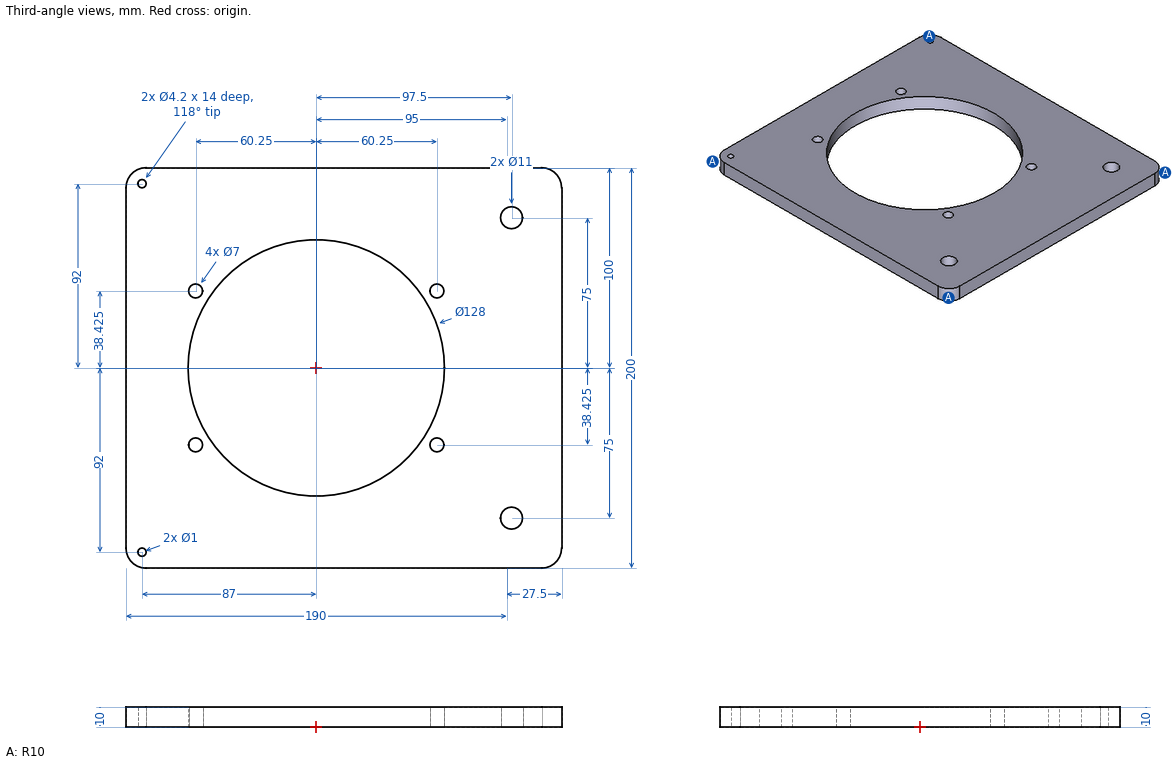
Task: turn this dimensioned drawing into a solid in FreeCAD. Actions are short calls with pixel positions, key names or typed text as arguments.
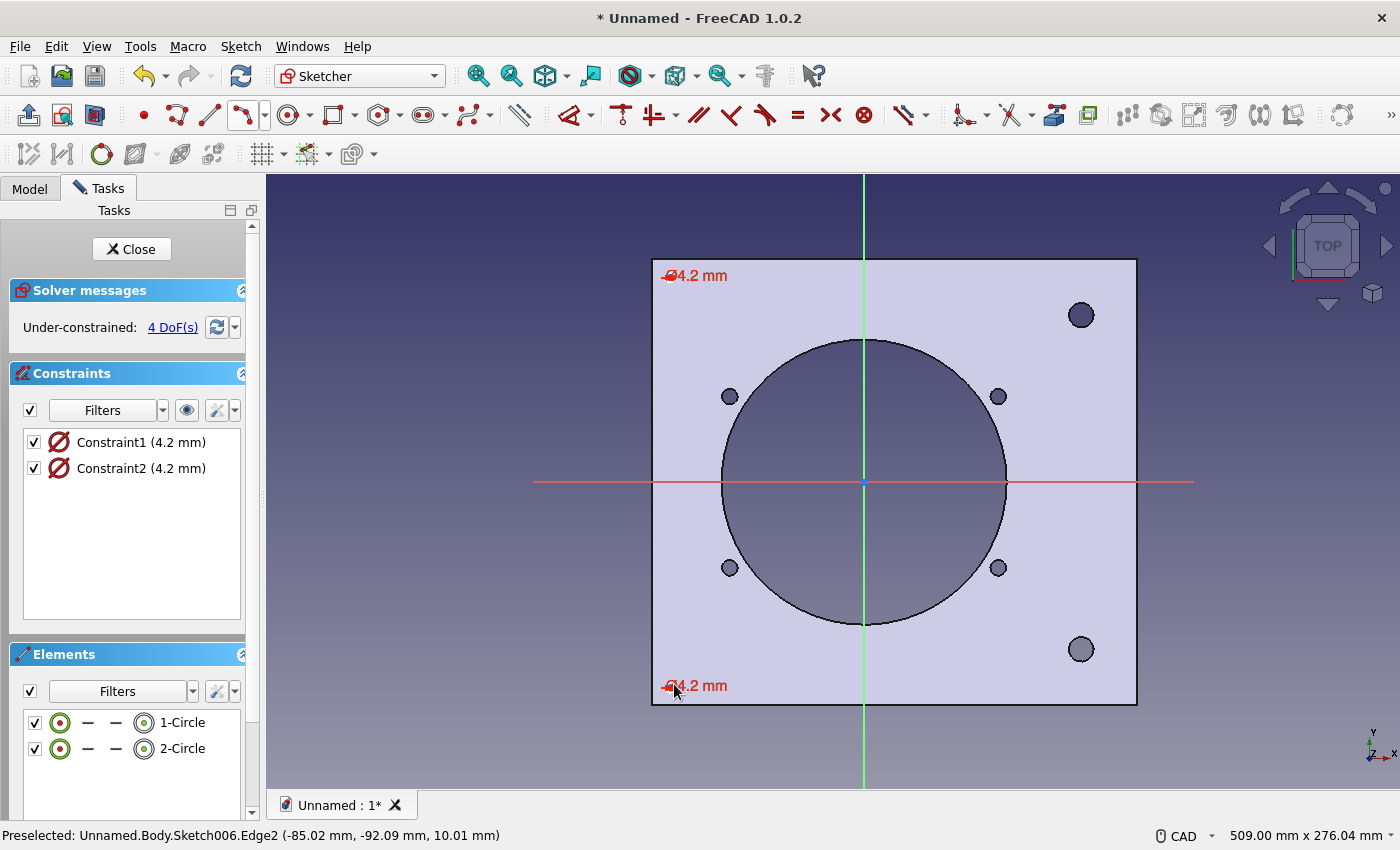
click(670, 278)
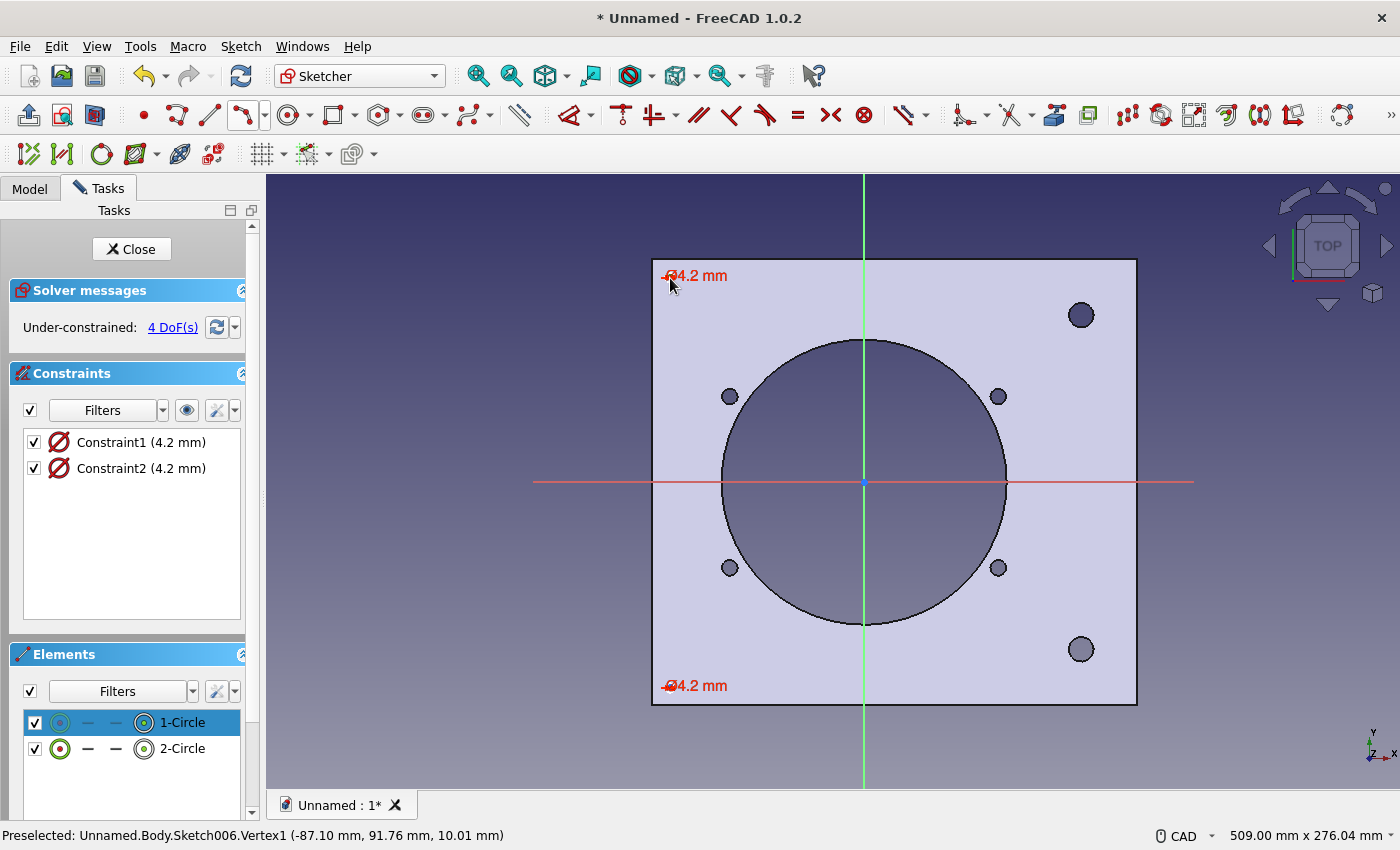
click(670, 688)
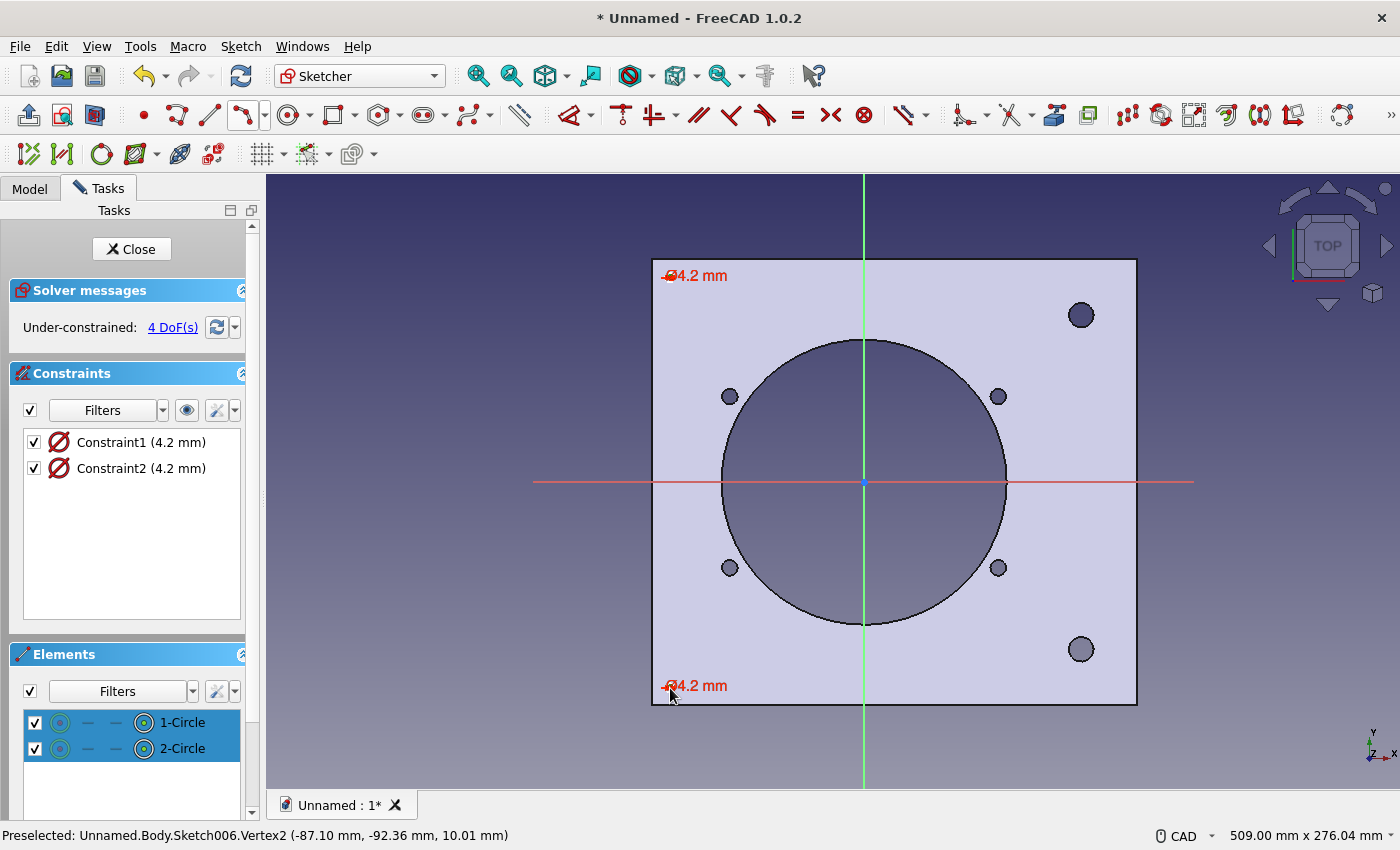
key(v)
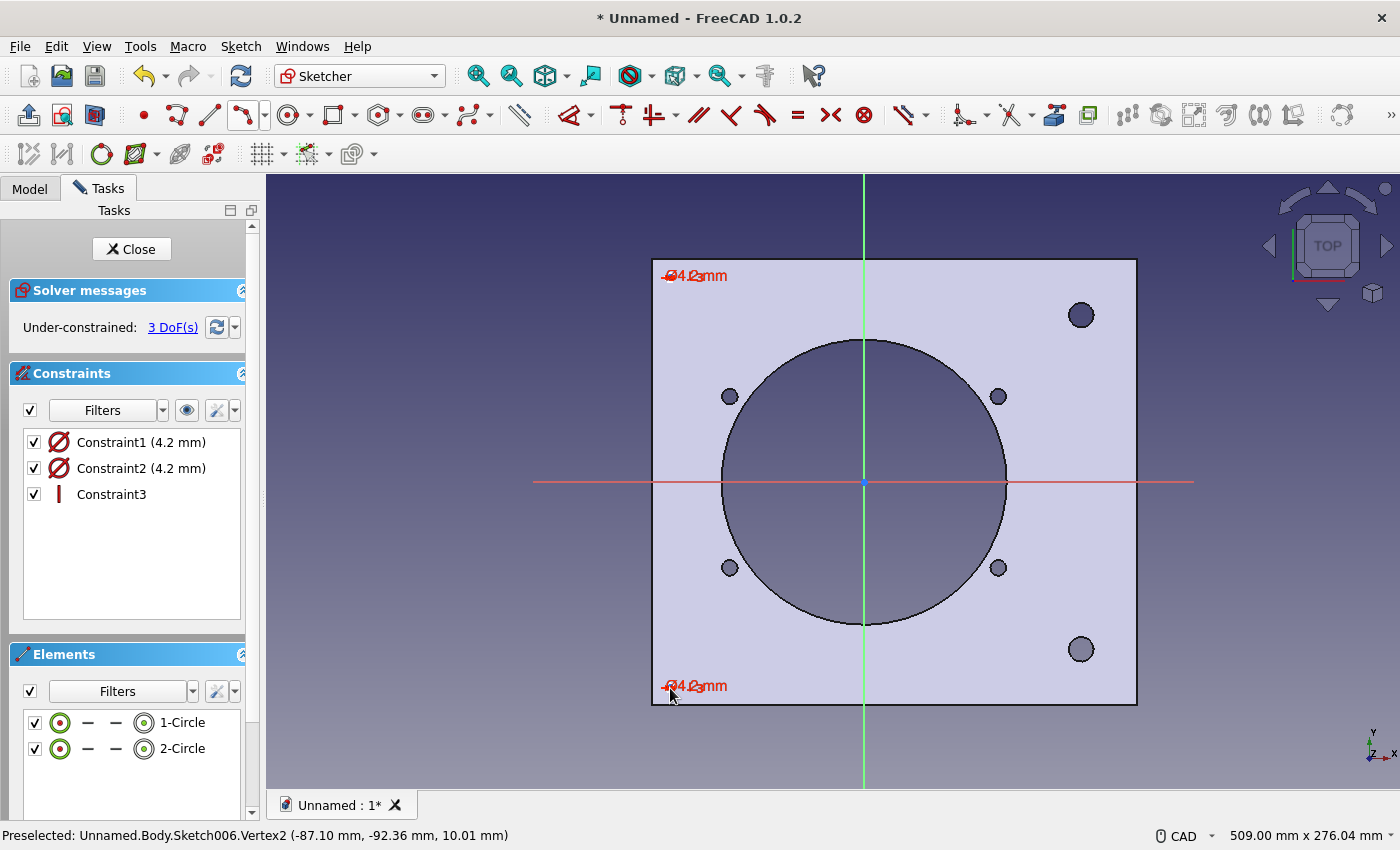
key(d)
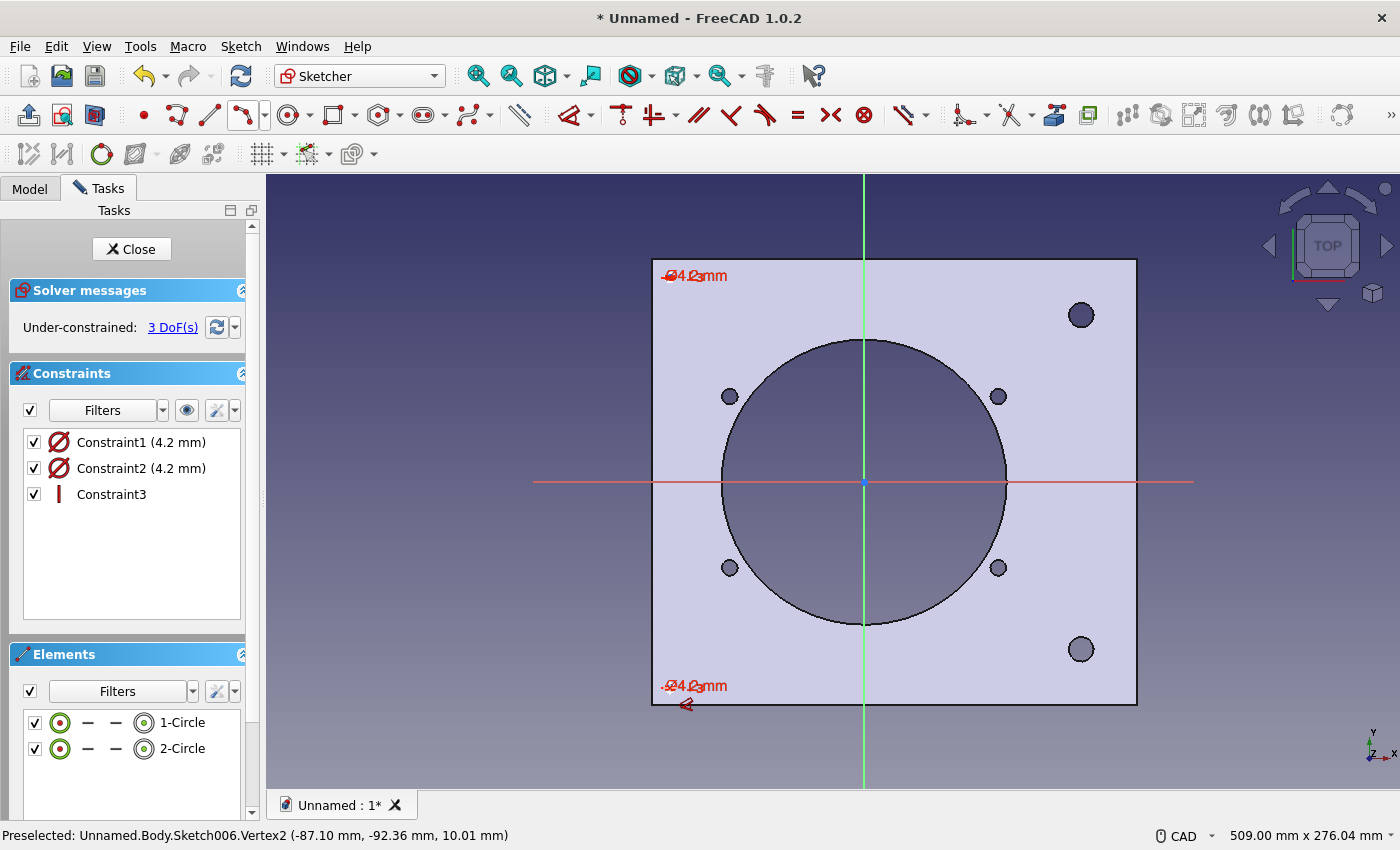
click(670, 278)
click(767, 244)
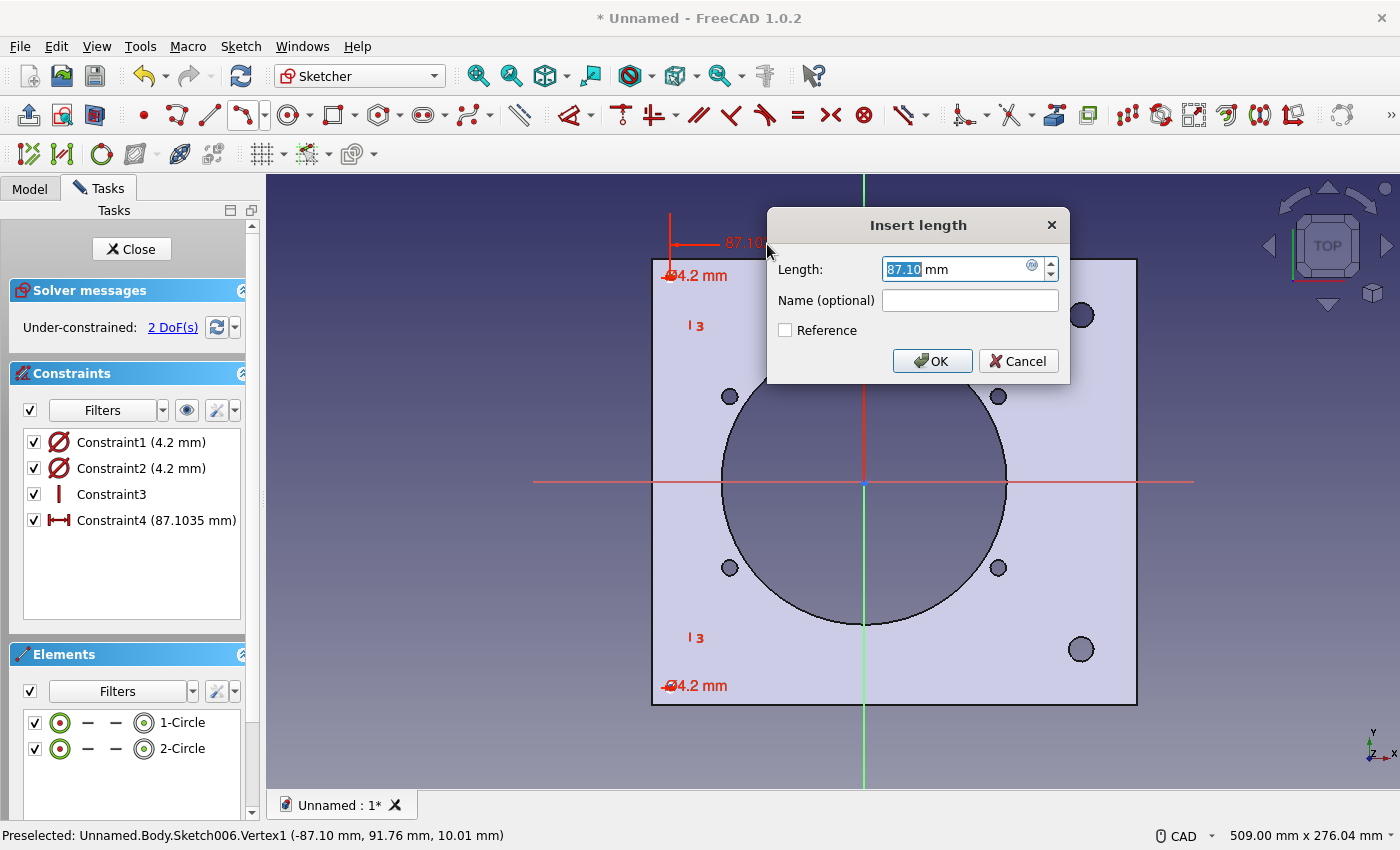
text(87)
key(Return)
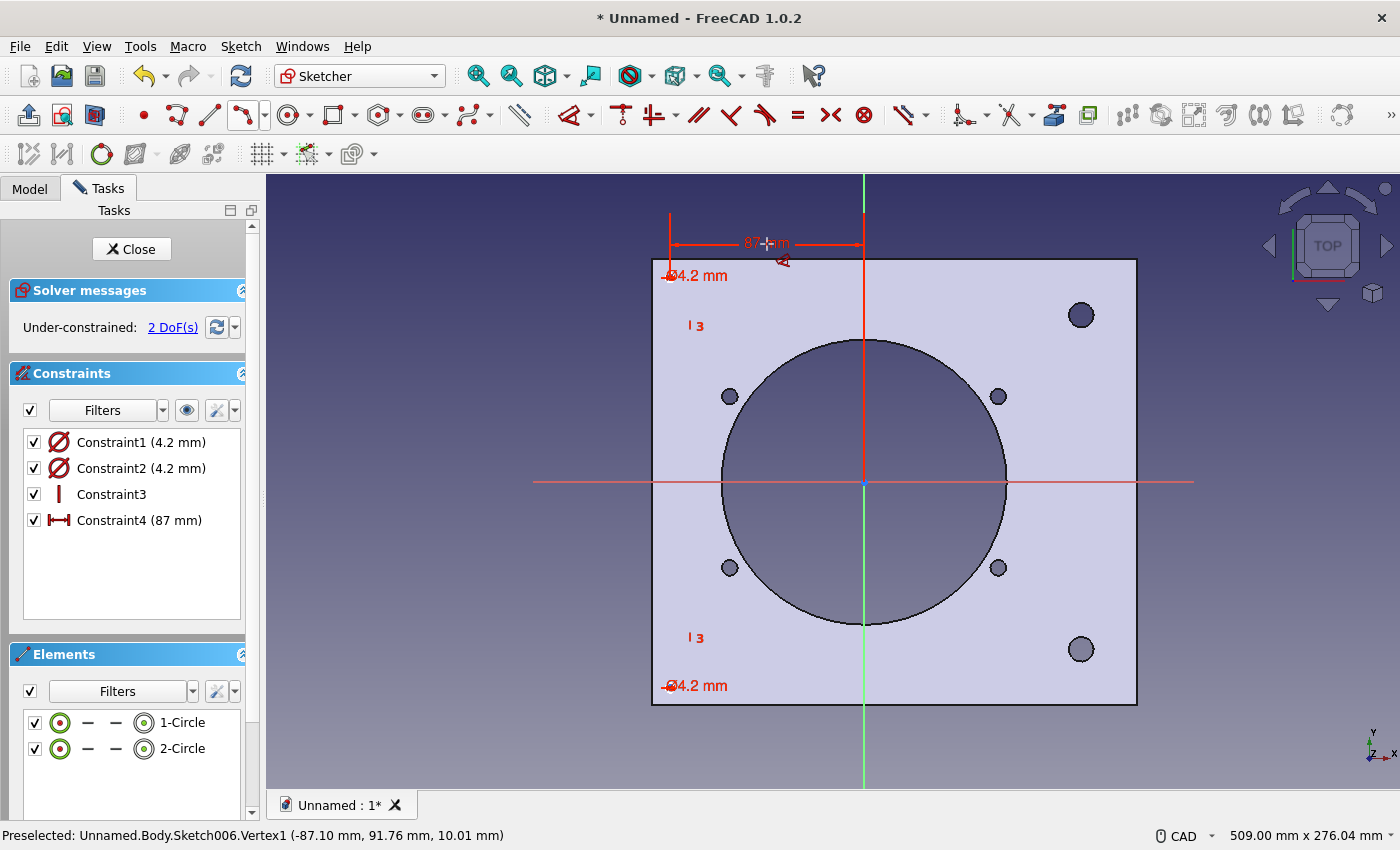
click(670, 278)
click(898, 380)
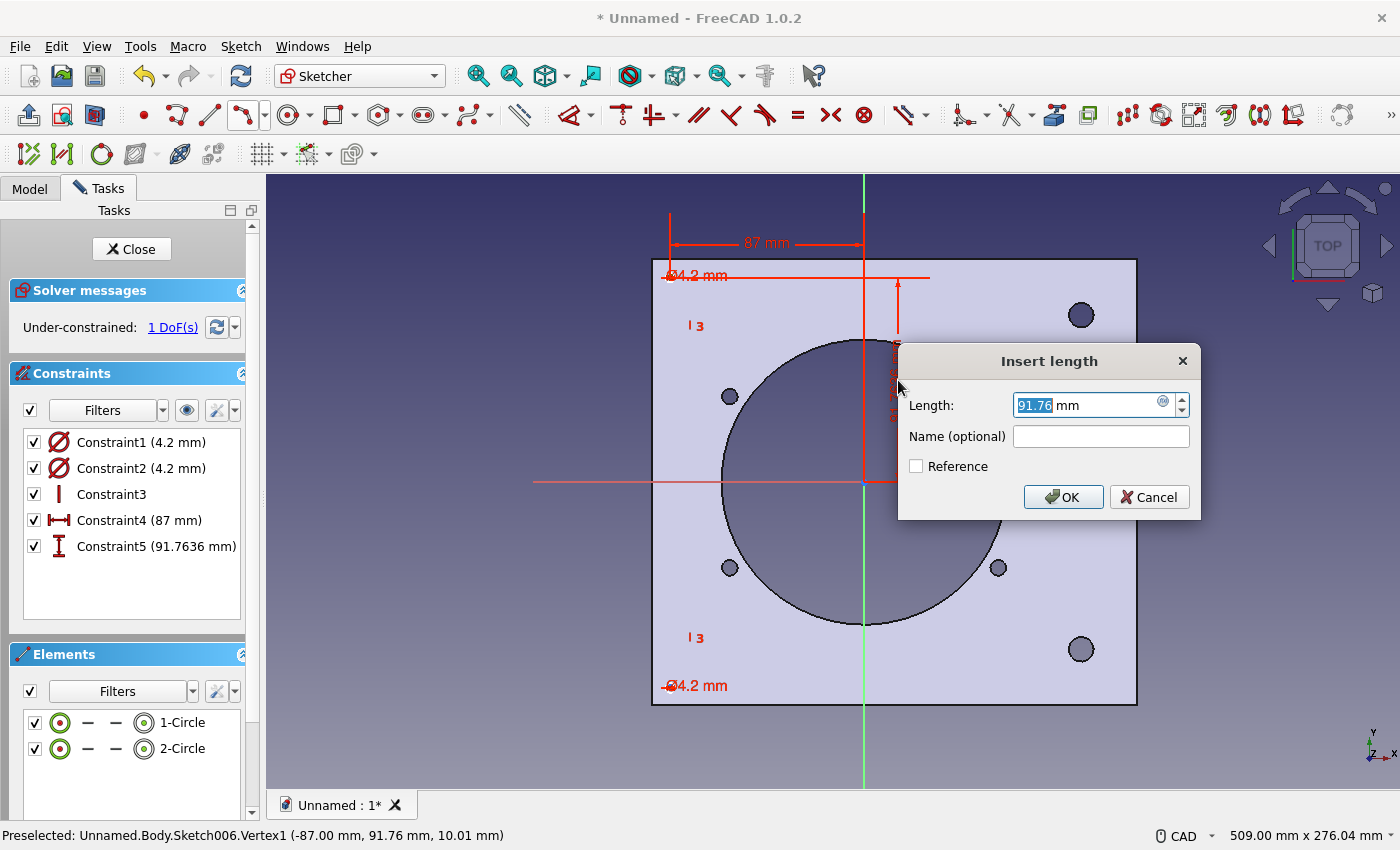
text(92)
key(Return)